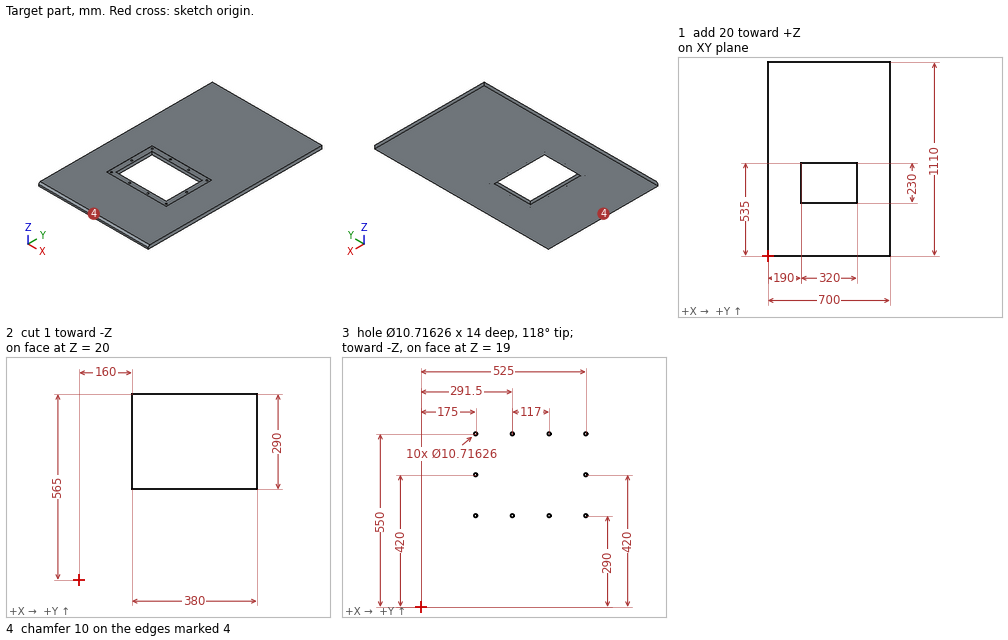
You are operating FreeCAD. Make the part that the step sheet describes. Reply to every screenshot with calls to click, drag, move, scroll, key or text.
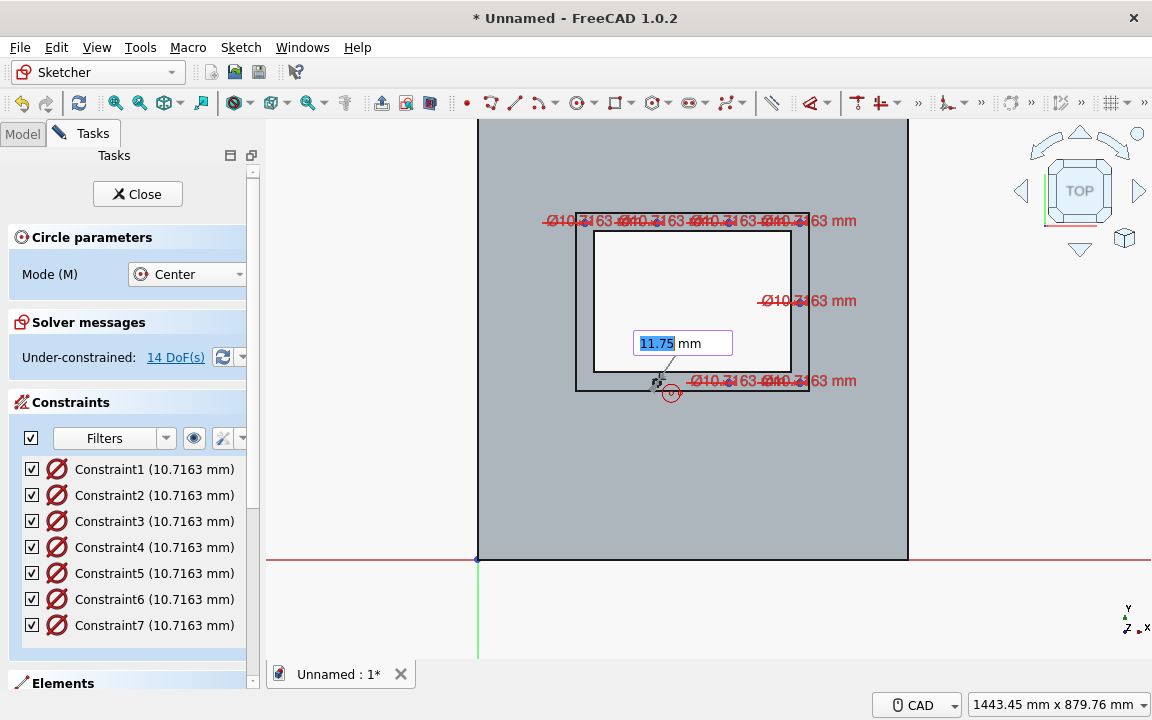
text(10.71626)
key(Return)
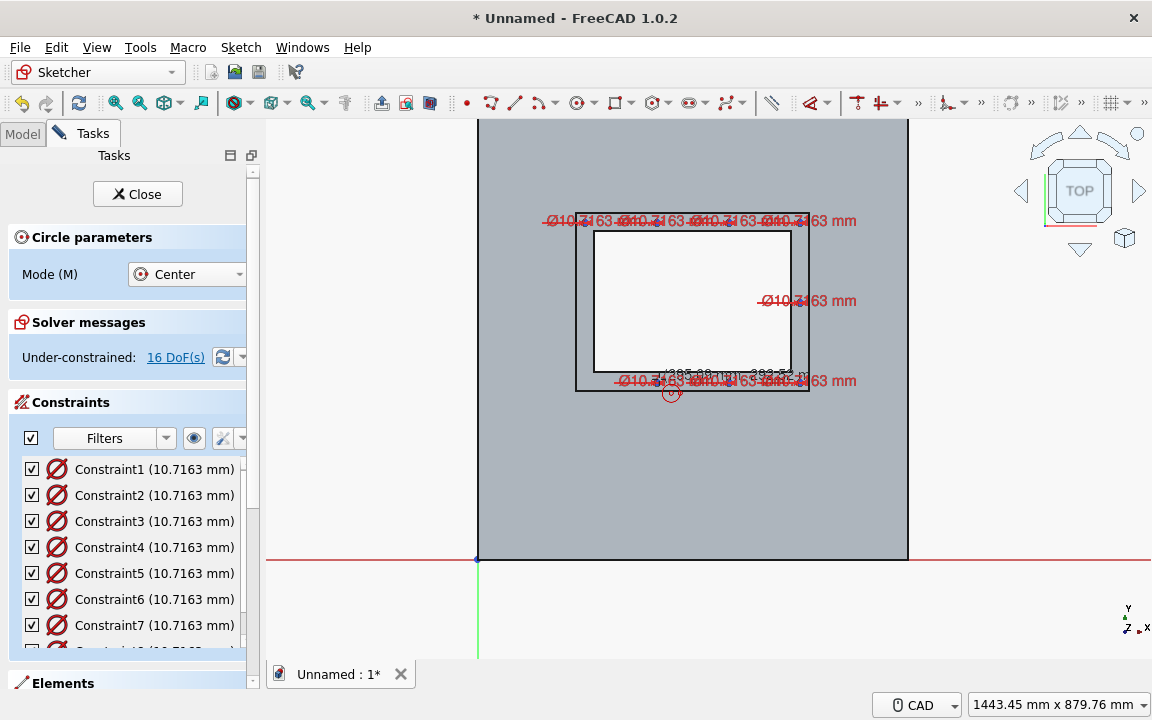
scroll(585, 382, up, 10)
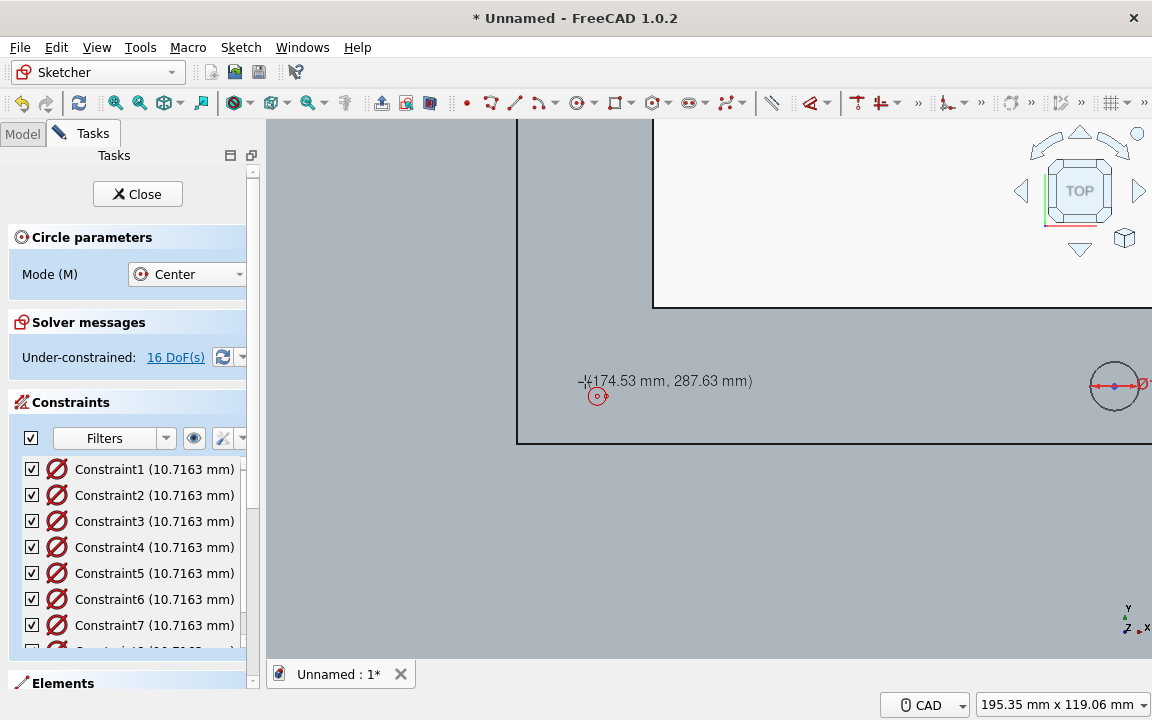
scroll(585, 382, down, 10)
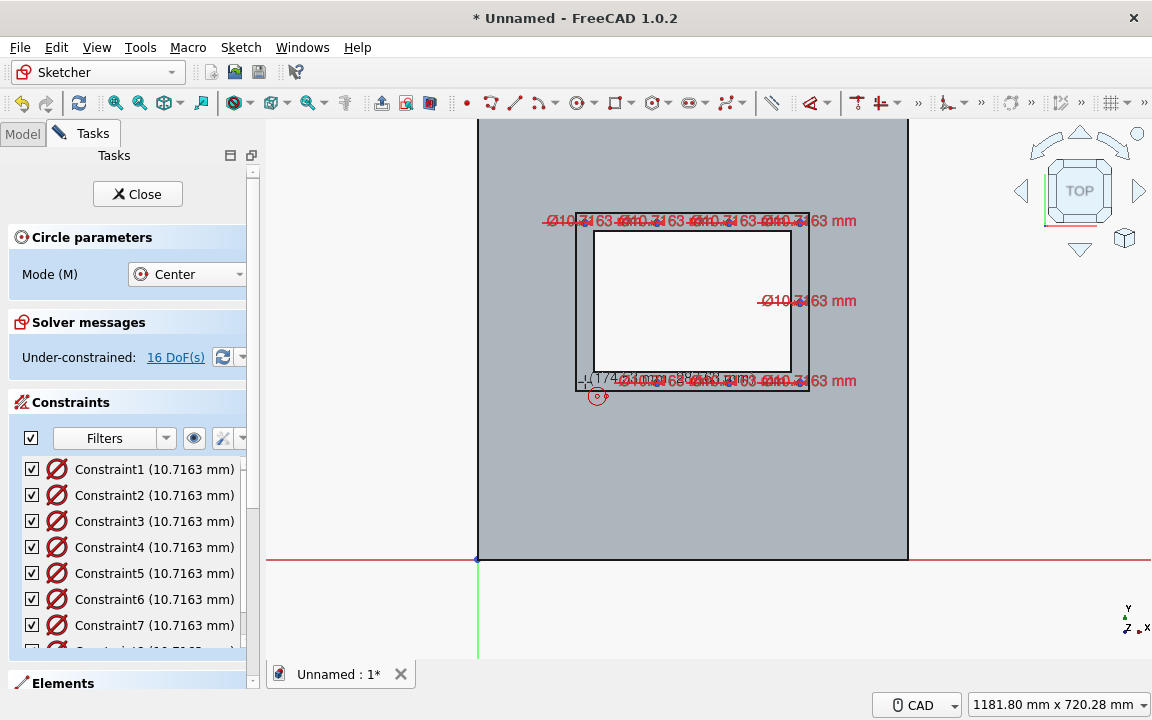
click(585, 382)
move(588, 379)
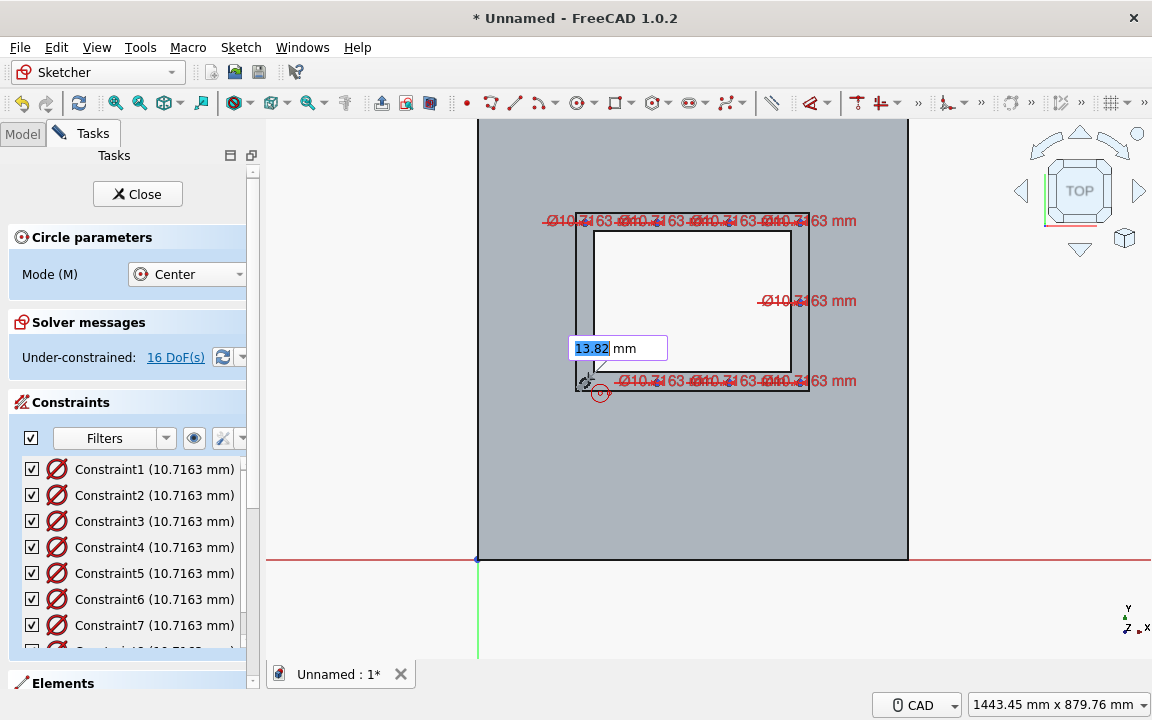
text(10.71626)
key(Return)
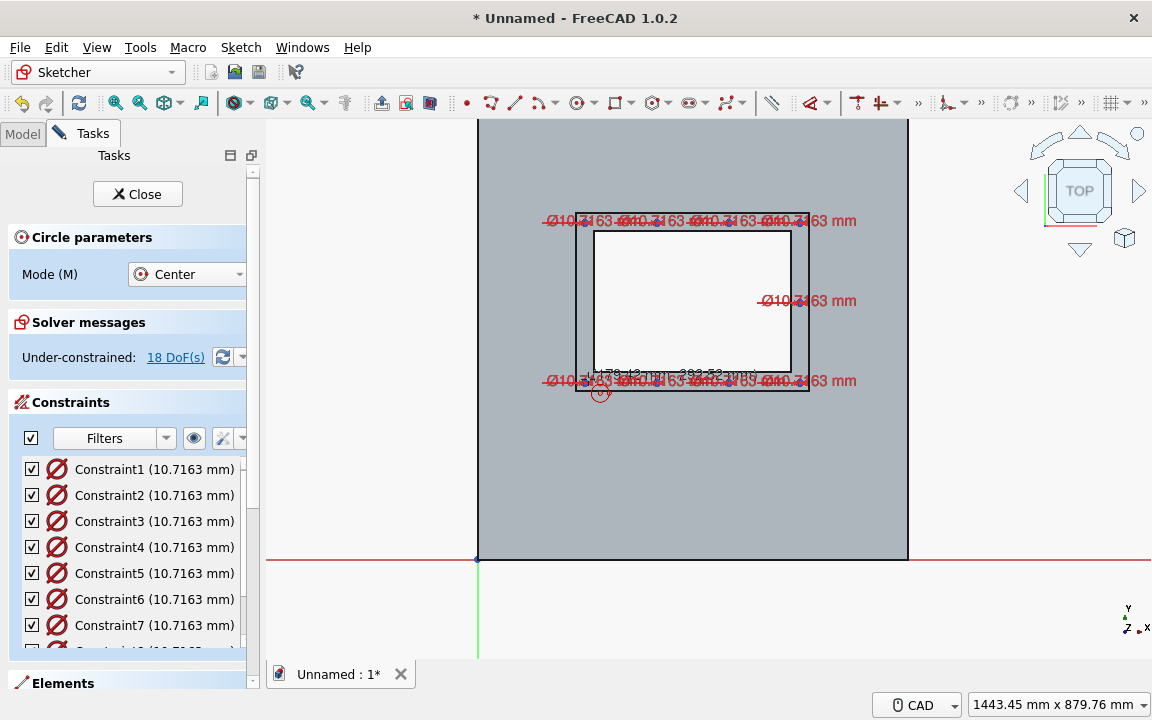
scroll(585, 302, up, 10)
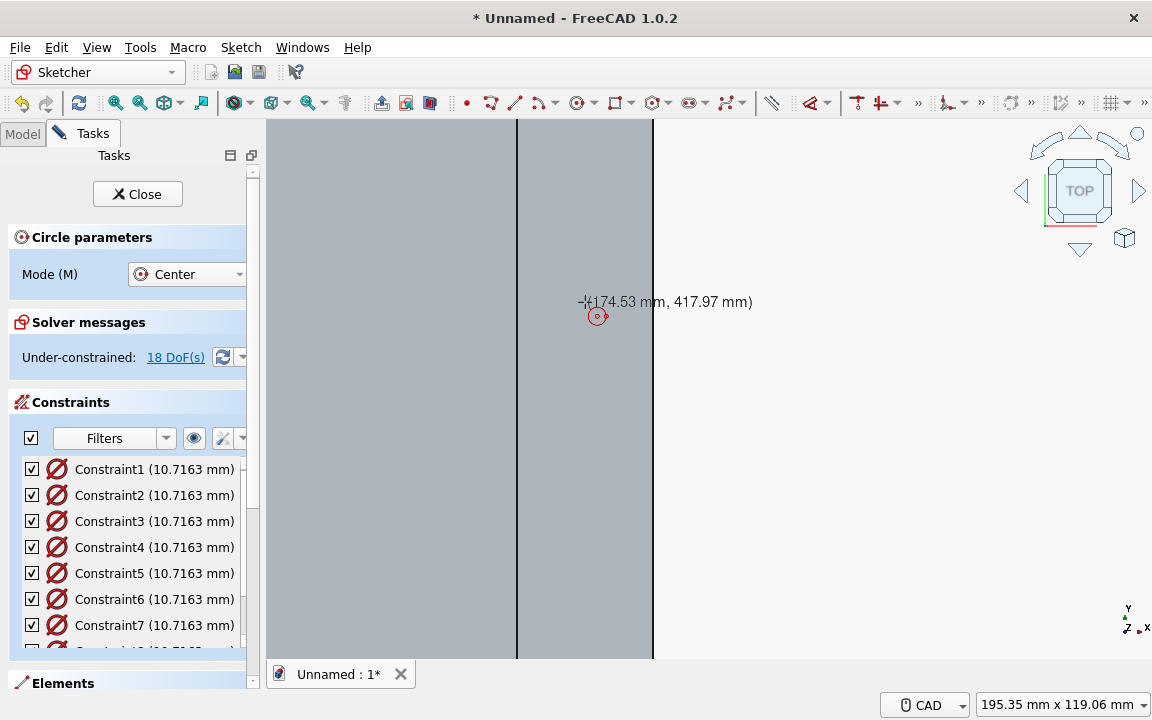
scroll(585, 302, down, 10)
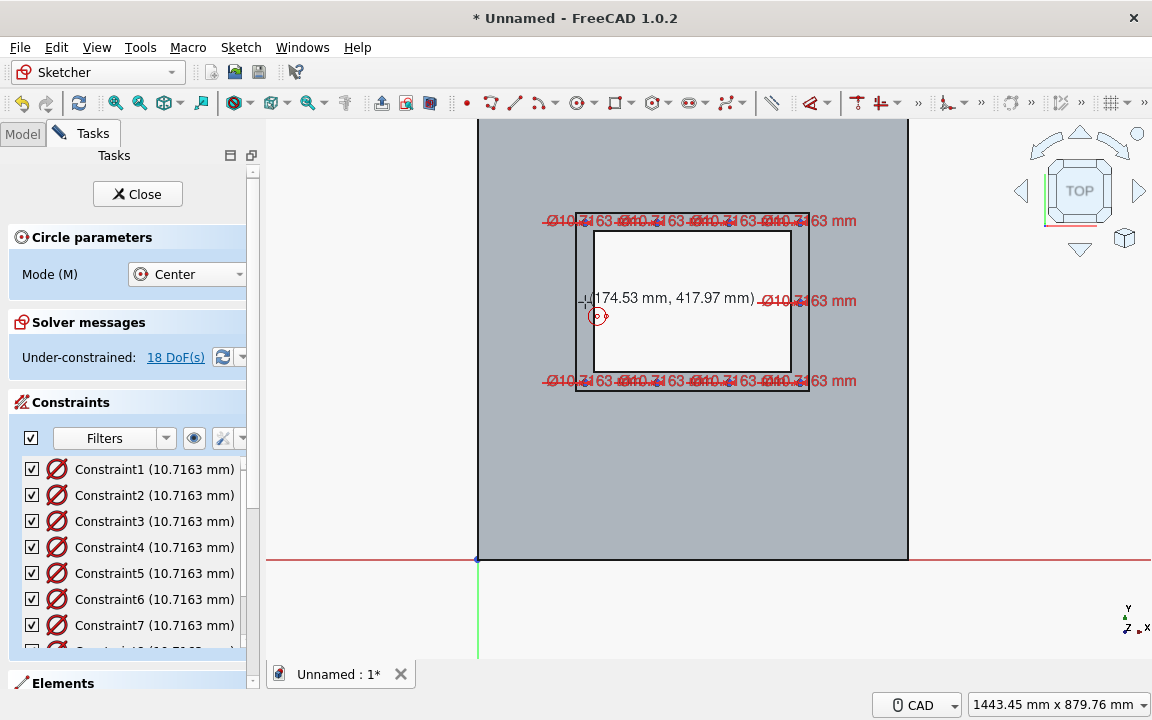
click(585, 302)
move(588, 299)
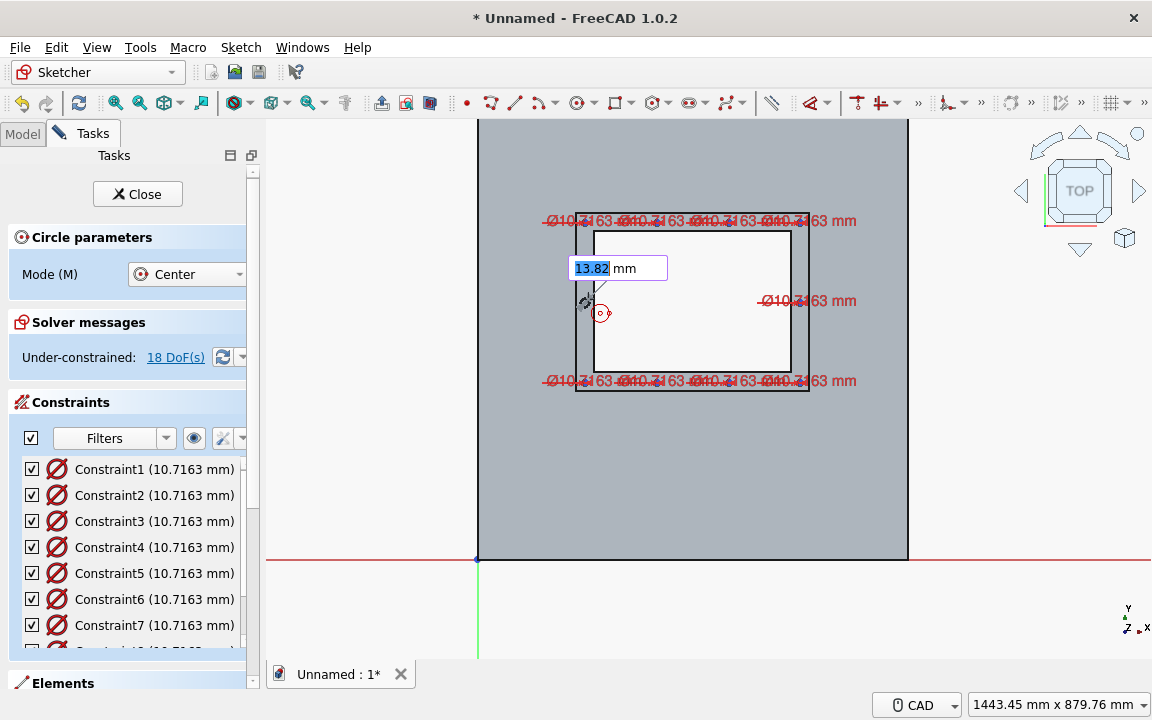
text(10.71626)
key(Return)
key(Escape)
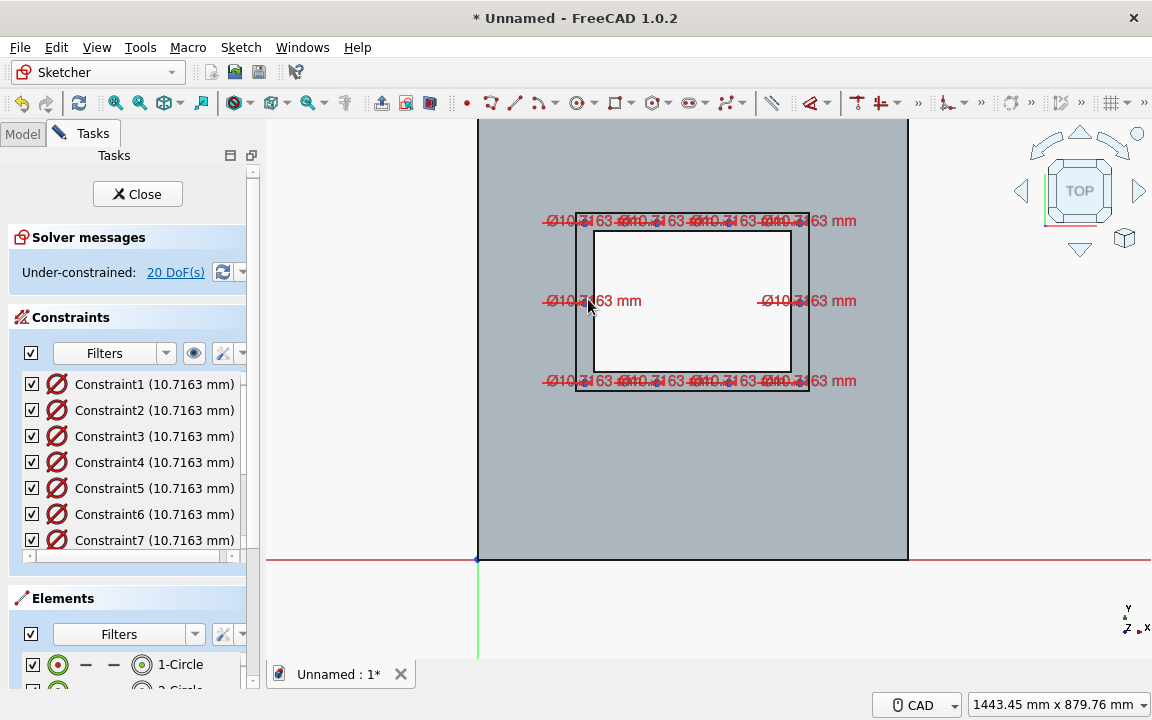
click(585, 223)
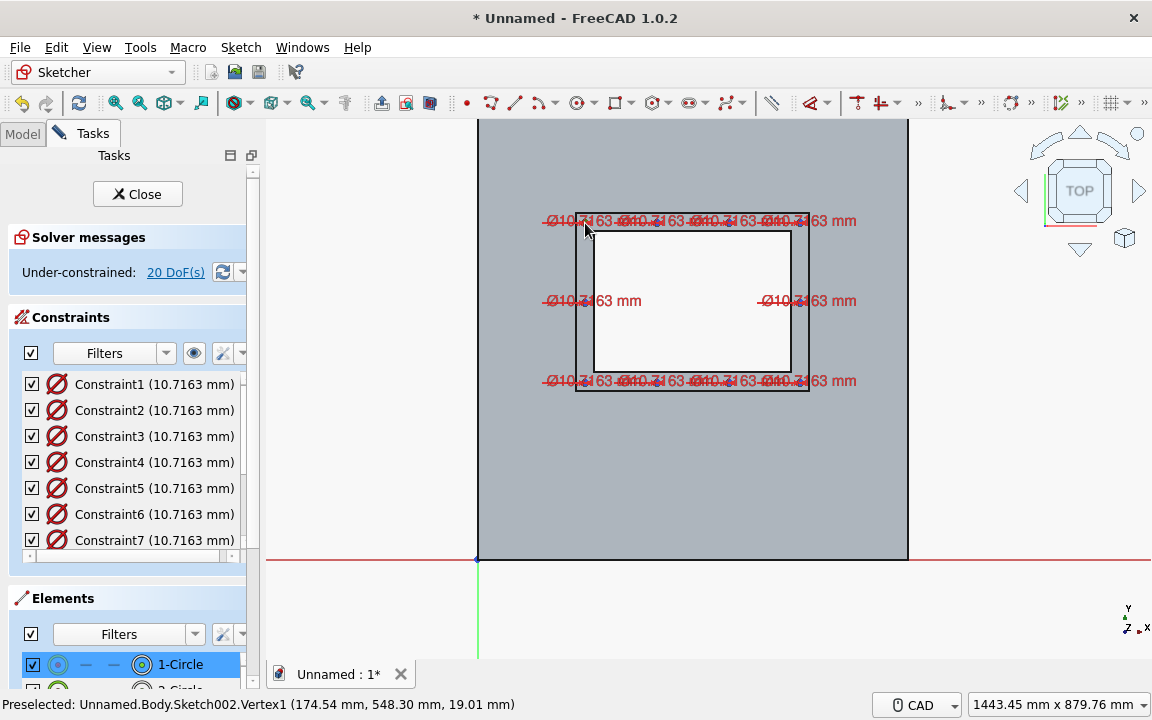
click(657, 223)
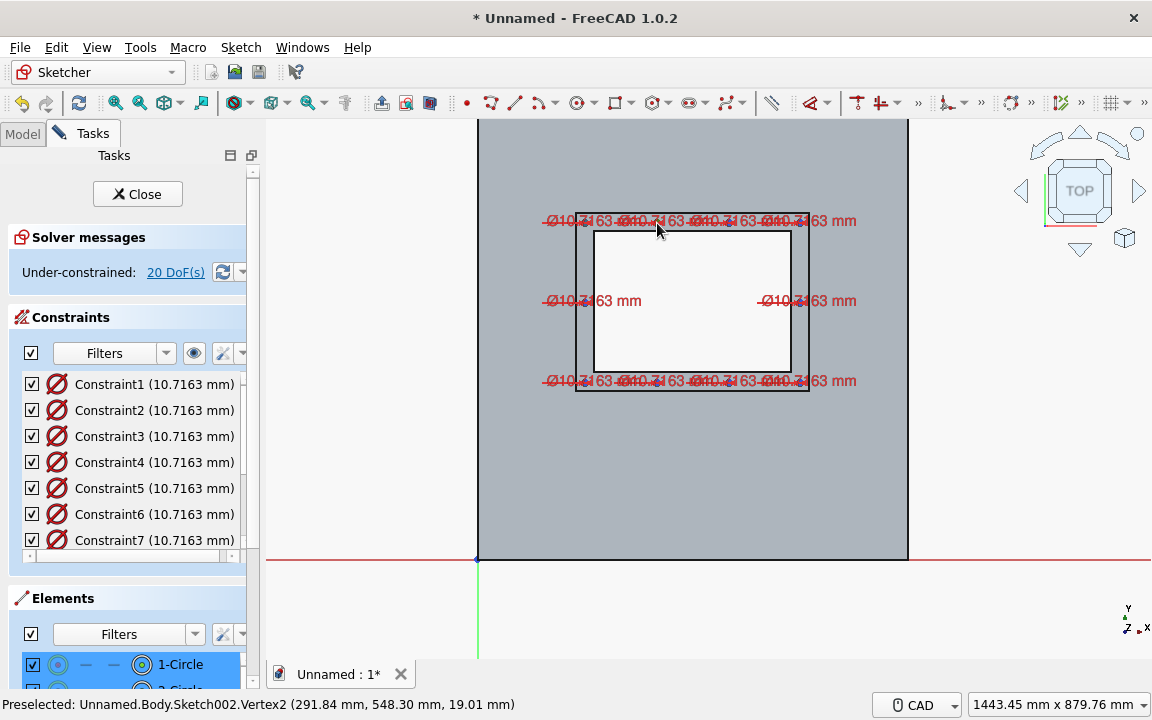
key(h)